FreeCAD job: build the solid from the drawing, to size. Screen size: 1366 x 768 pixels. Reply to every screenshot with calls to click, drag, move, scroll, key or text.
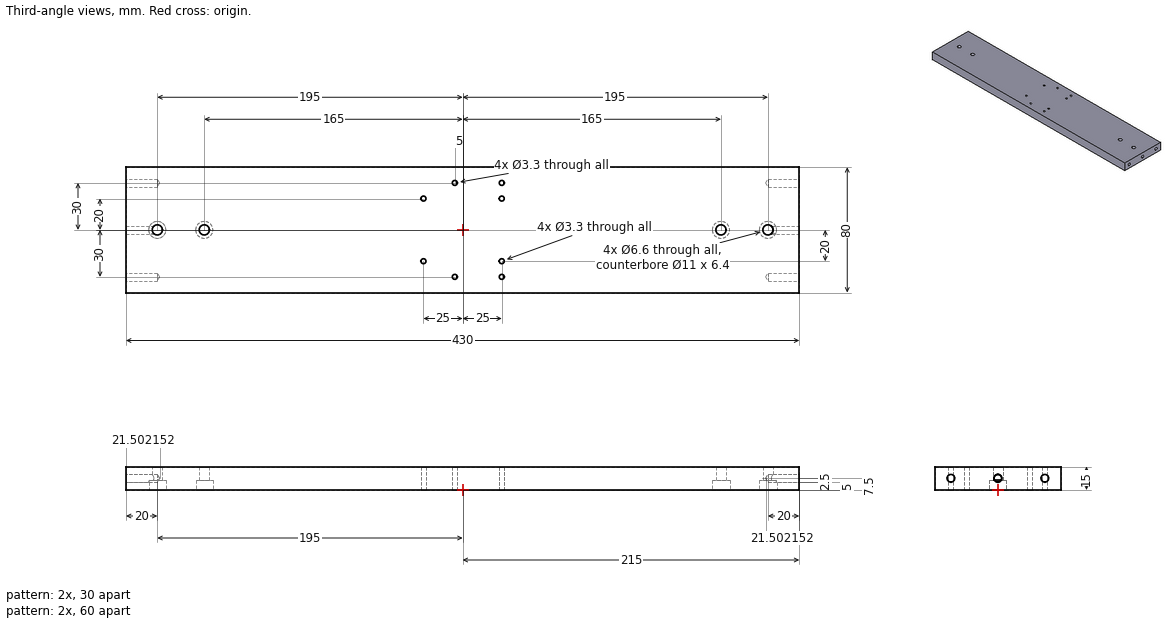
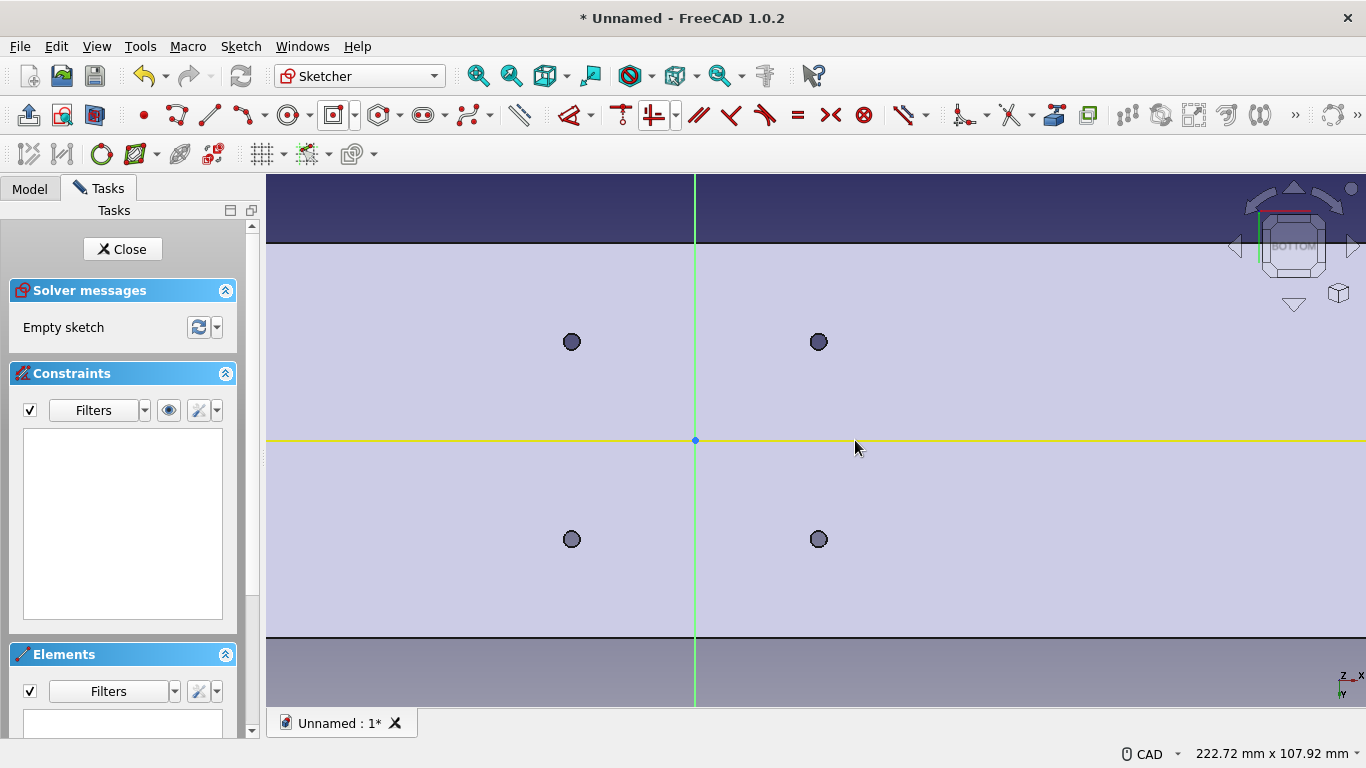
click(288, 116)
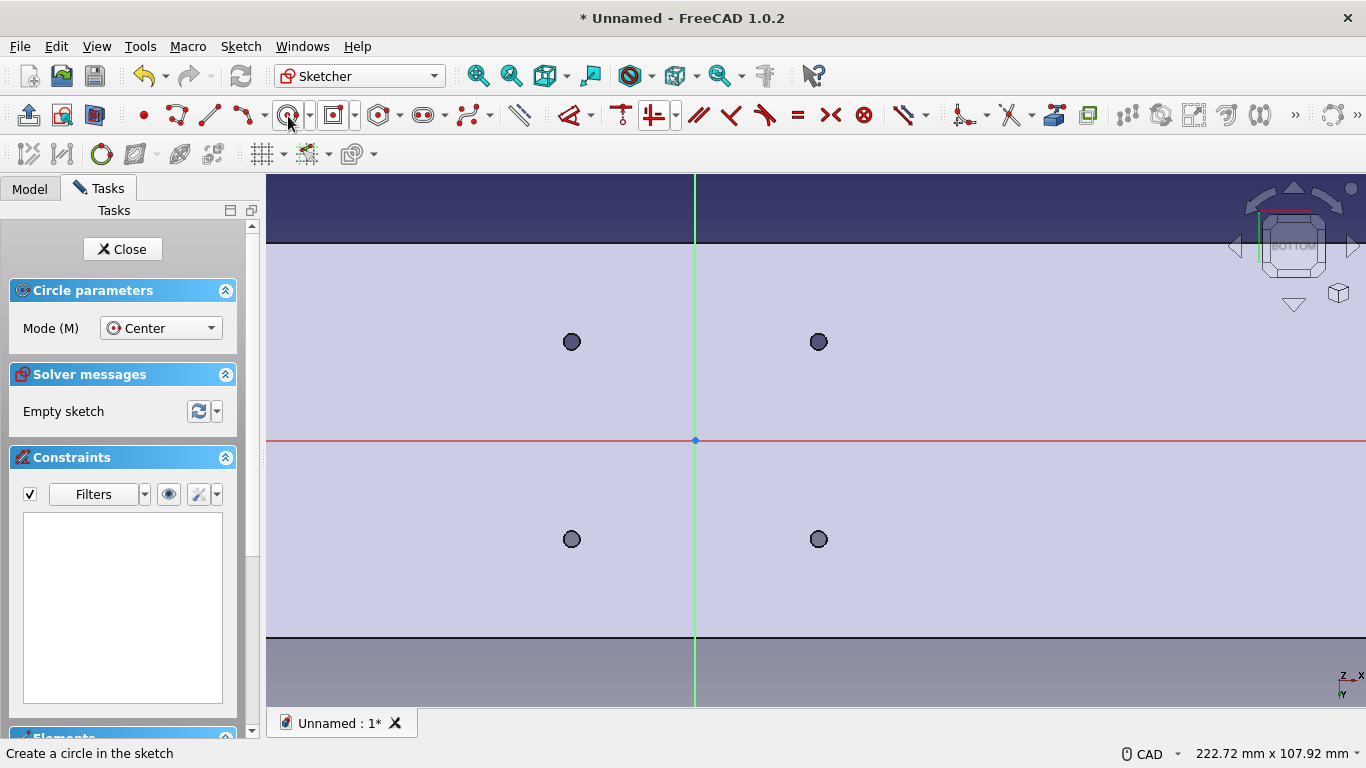
scroll(671, 589, up, 6)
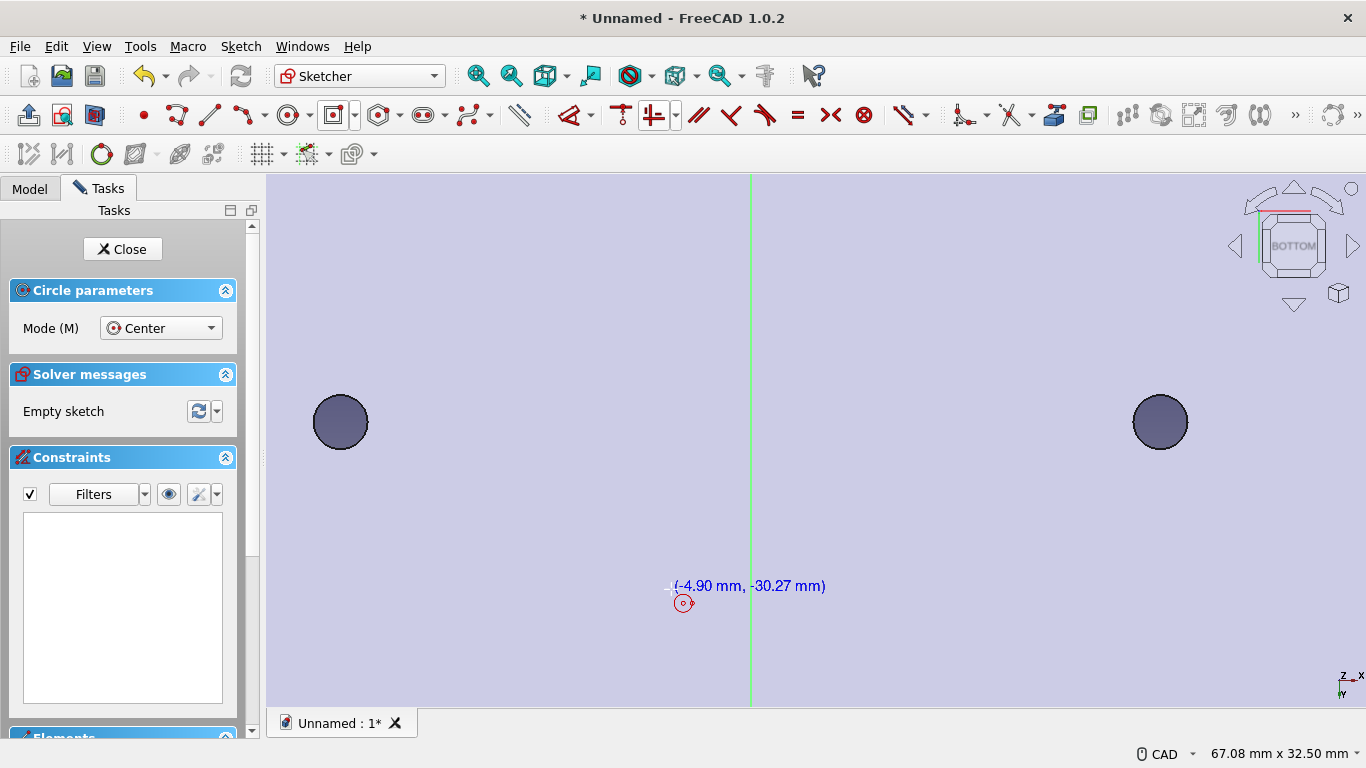
click(669, 586)
click(688, 567)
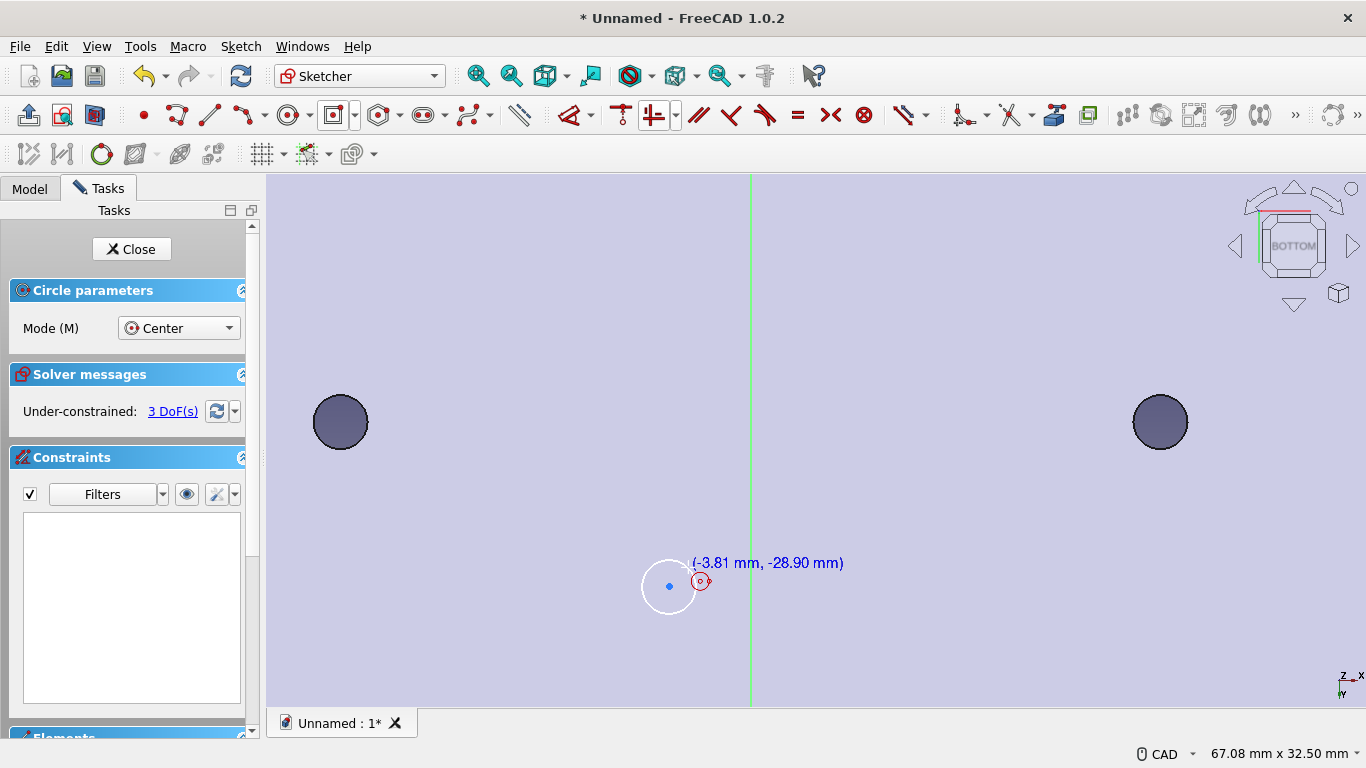
scroll(676, 590, down, 6)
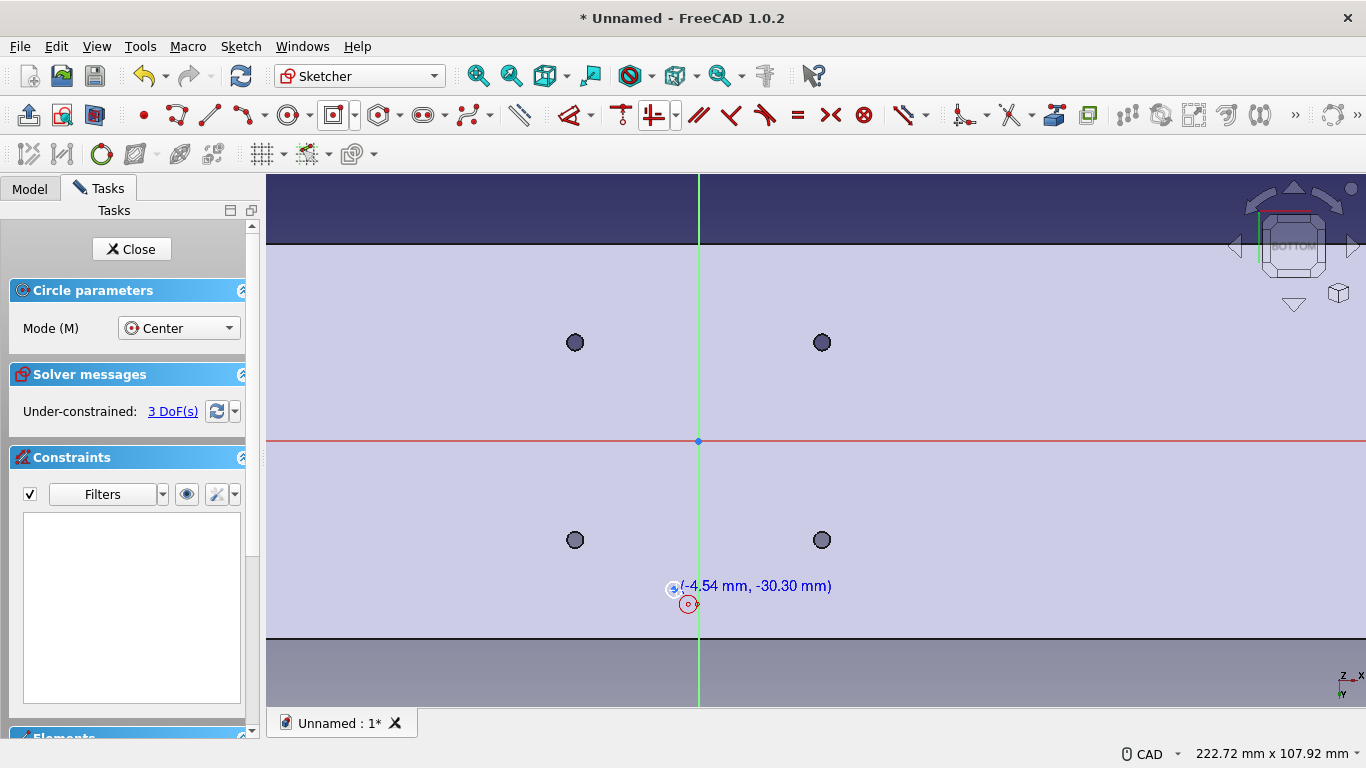
scroll(674, 293, up, 6)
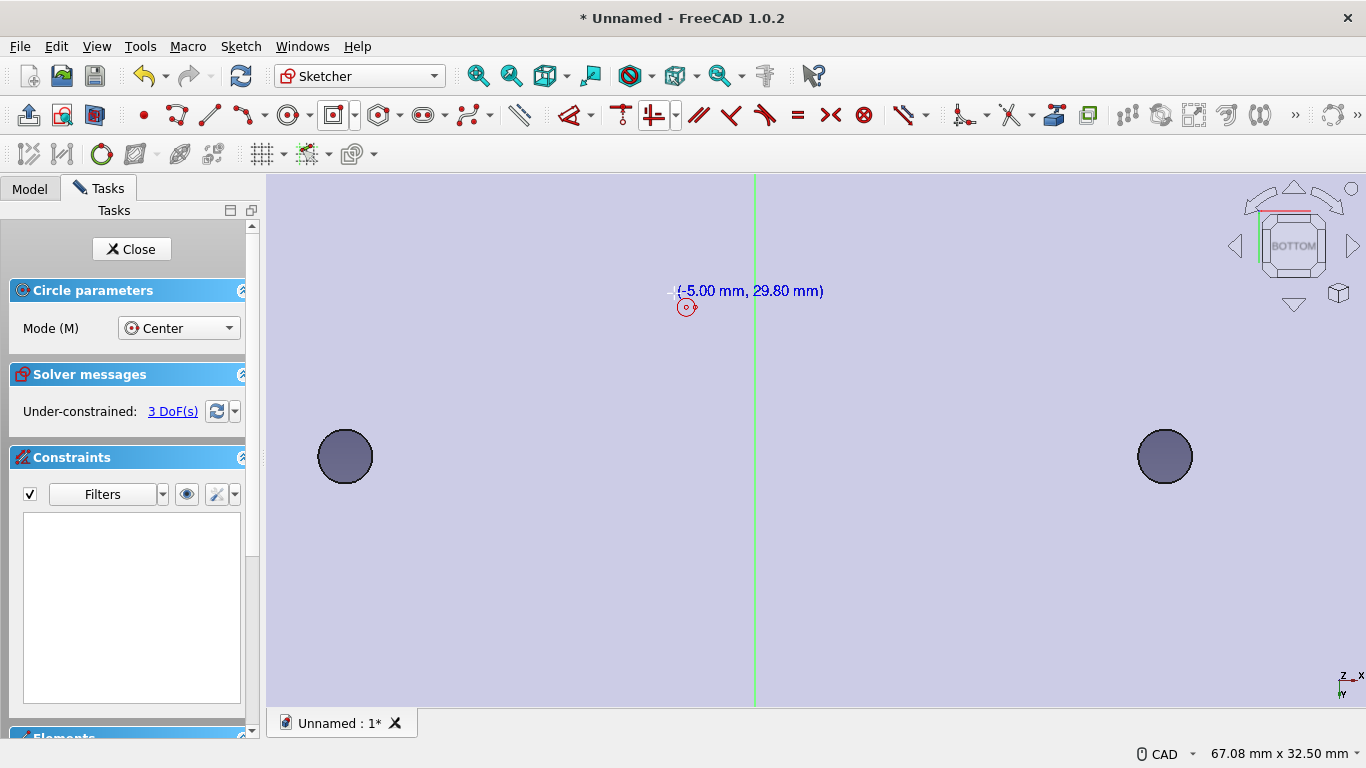
click(673, 293)
click(692, 273)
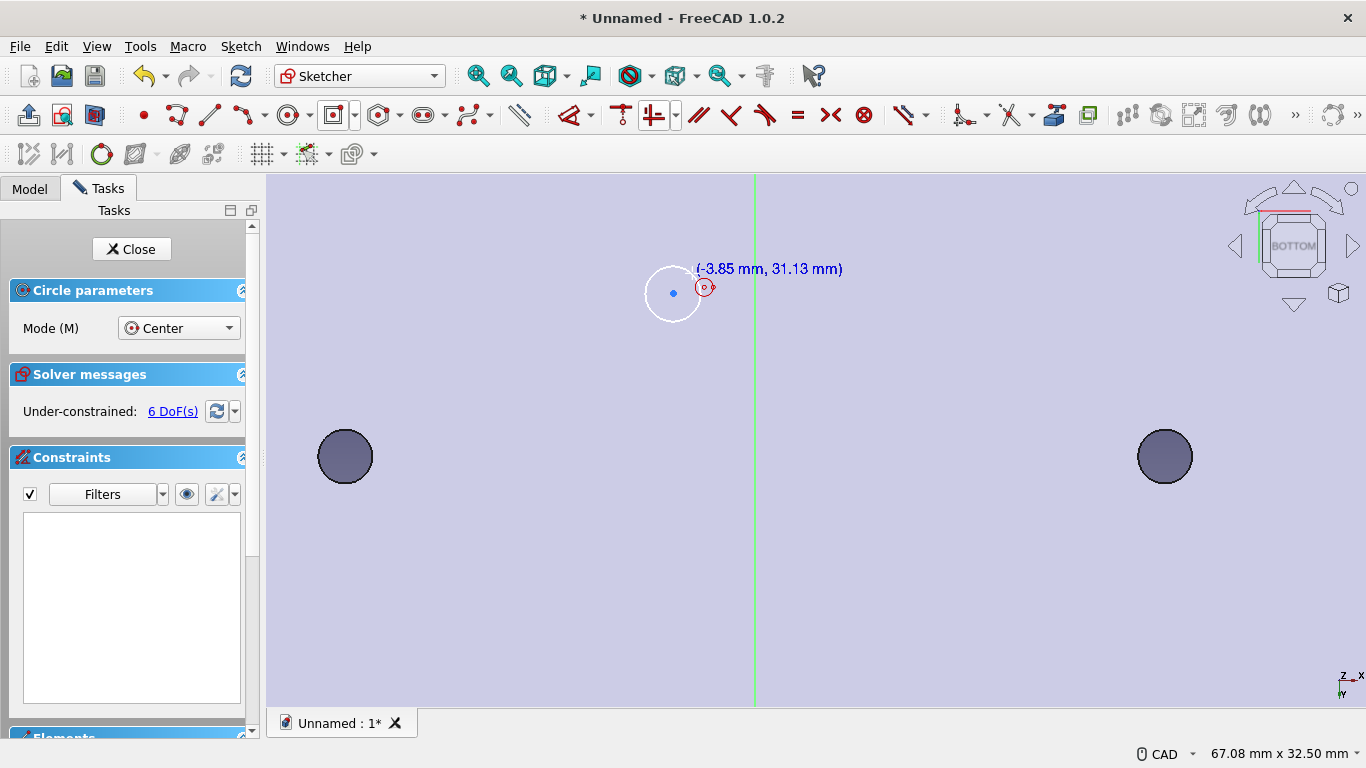
scroll(674, 292, down, 6)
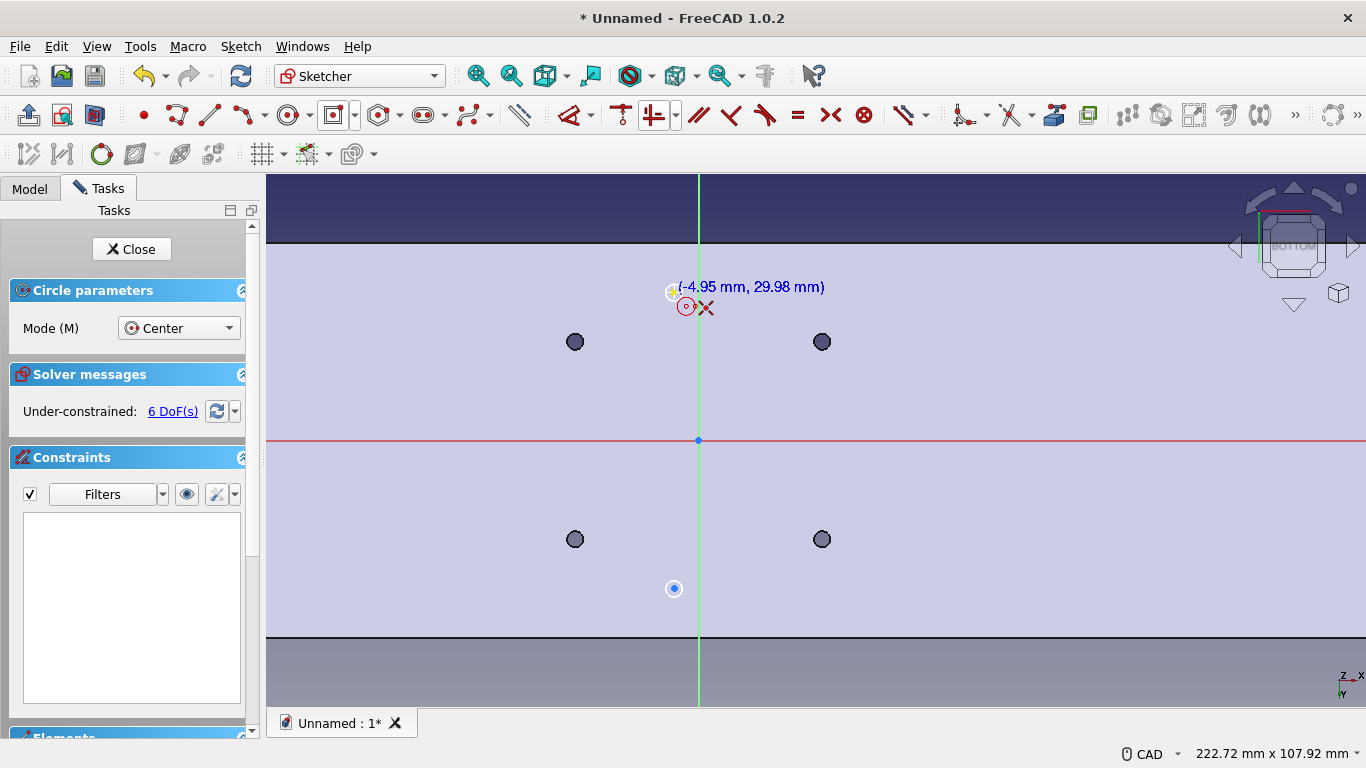
scroll(822, 589, up, 6)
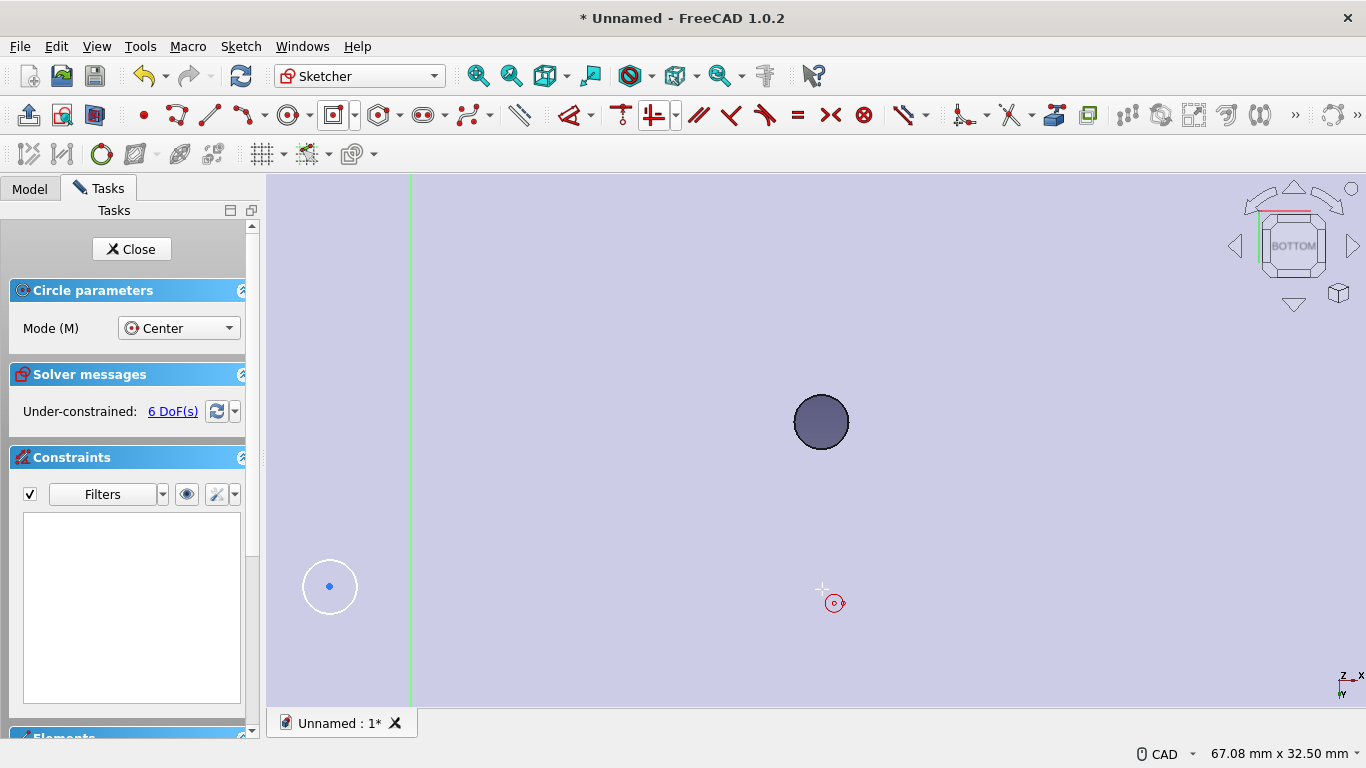
click(821, 586)
click(841, 567)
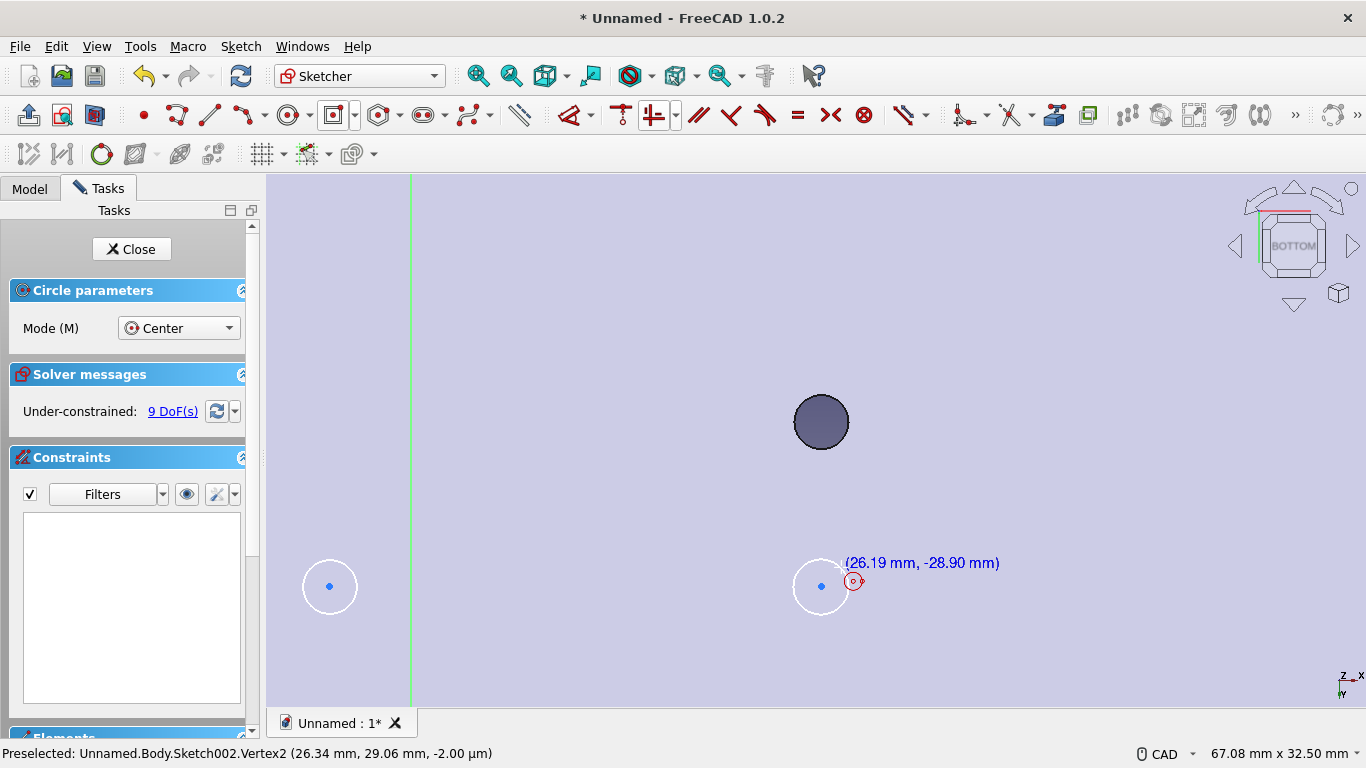
scroll(822, 590, down, 6)